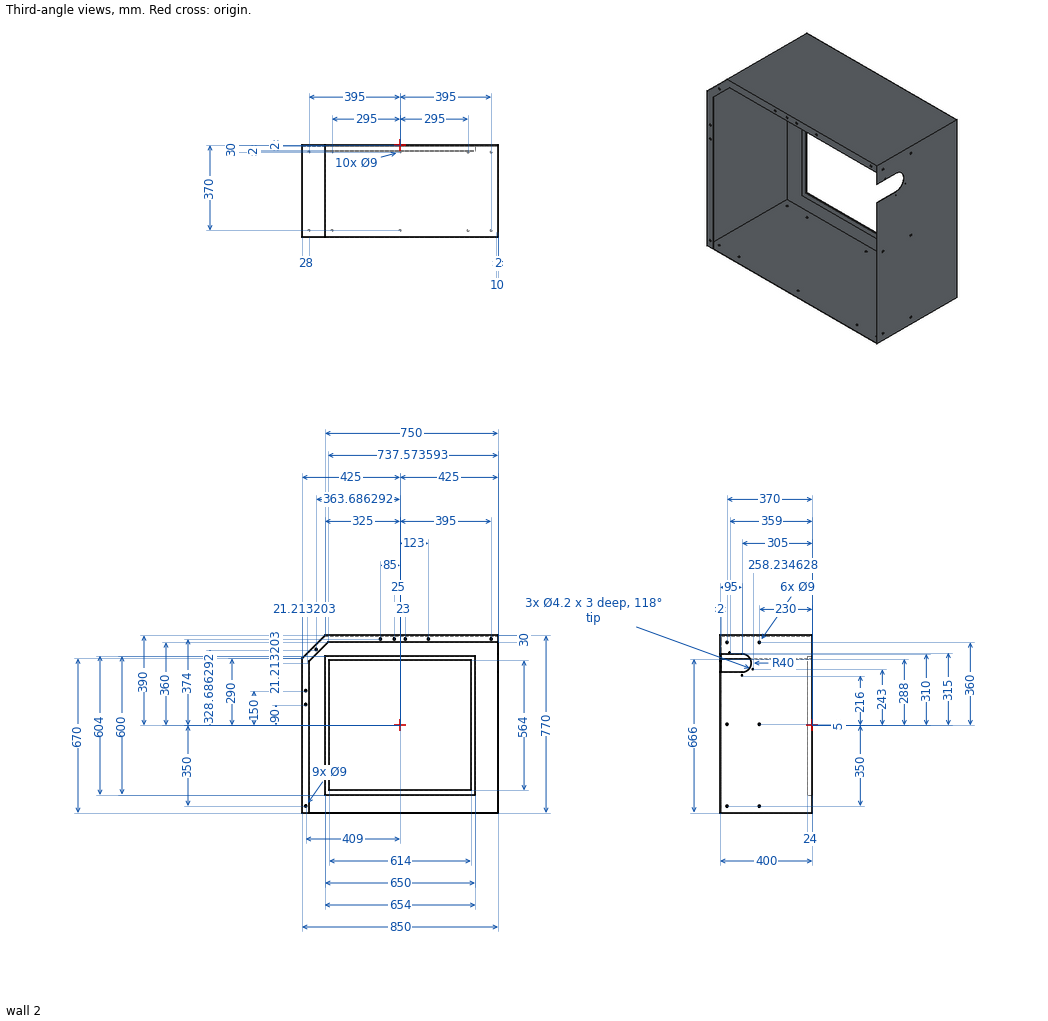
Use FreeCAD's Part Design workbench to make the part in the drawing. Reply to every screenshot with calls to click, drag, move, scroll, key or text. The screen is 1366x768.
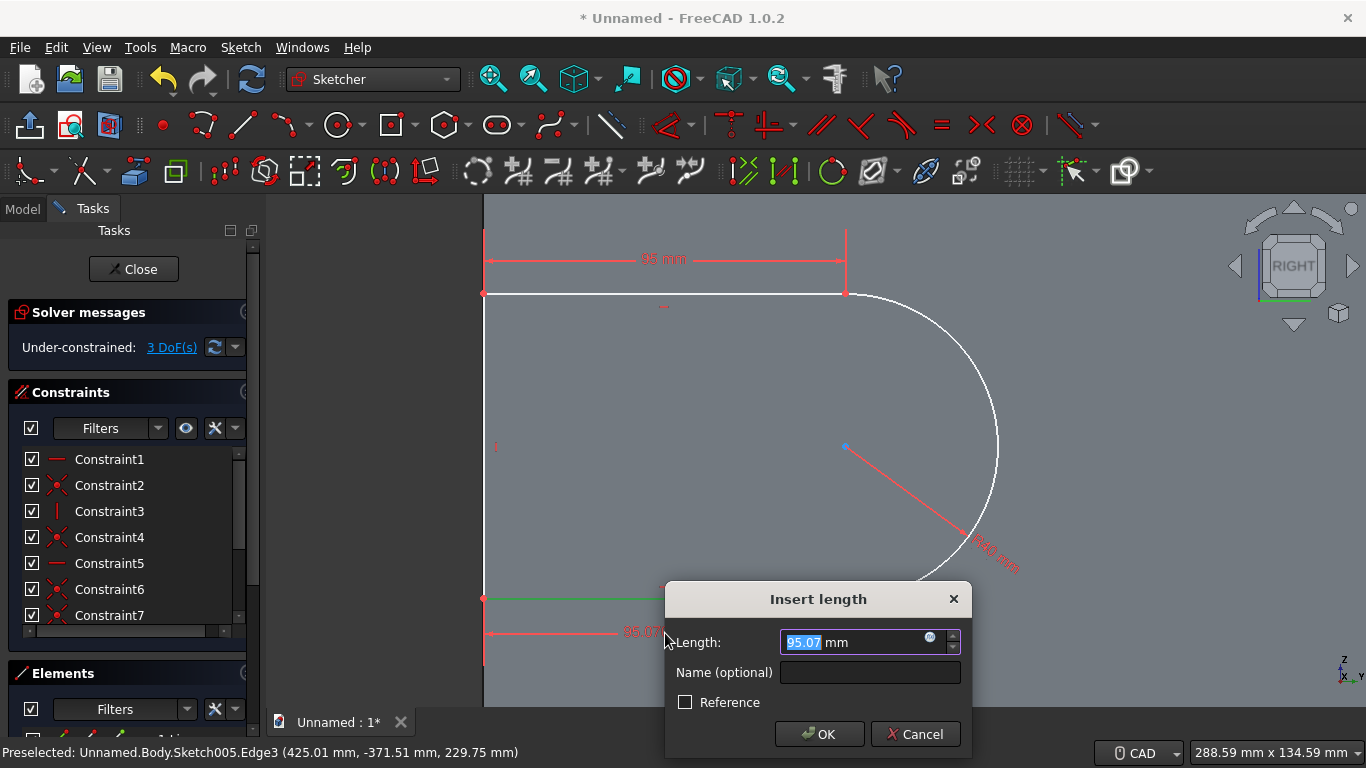
text(95)
key(Return)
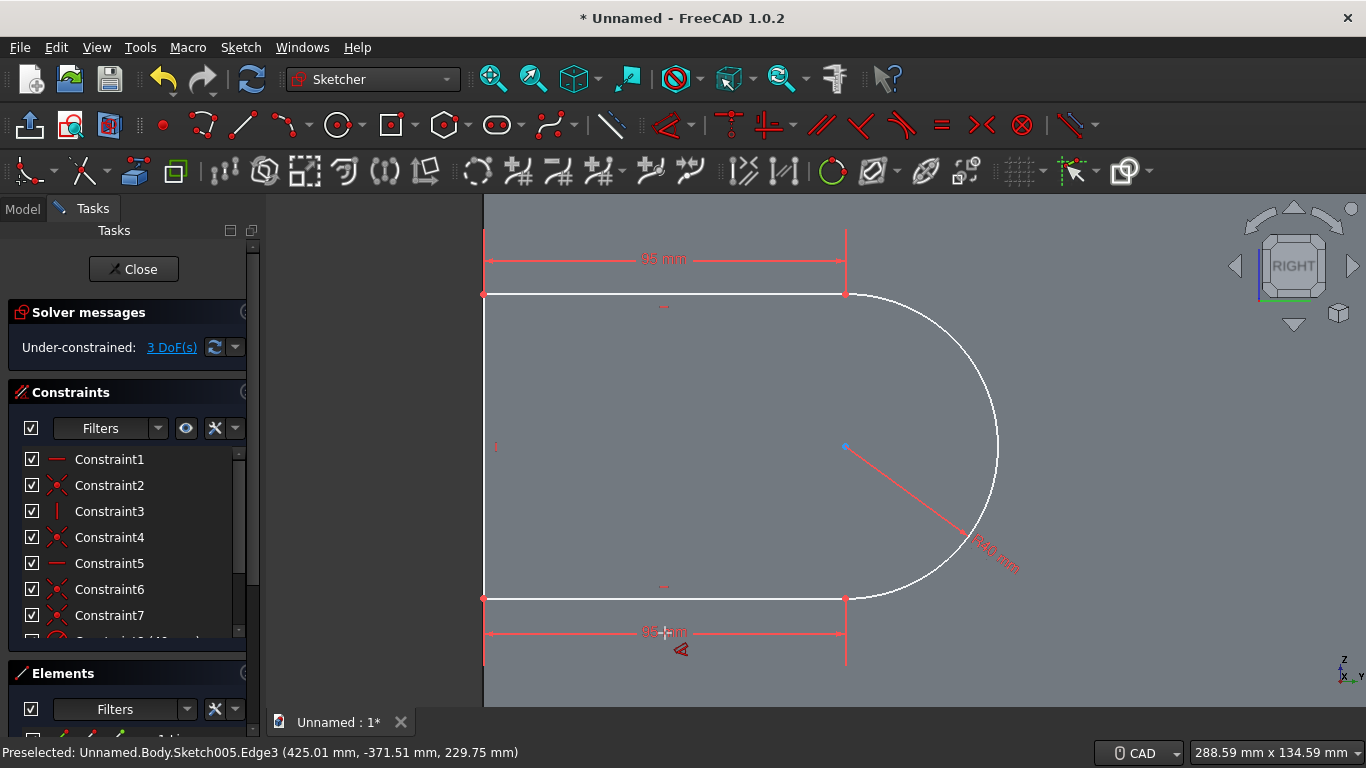
click(846, 294)
click(1023, 260)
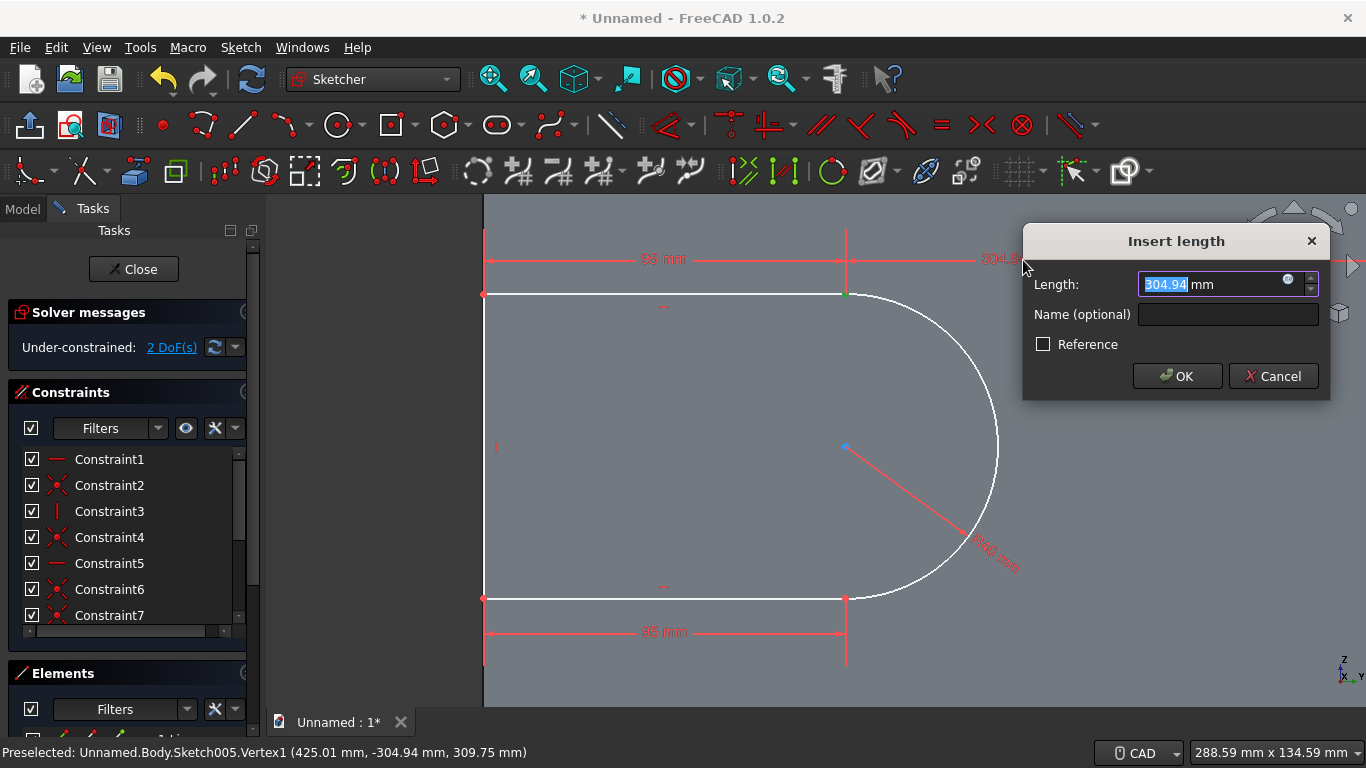
text(305)
key(Return)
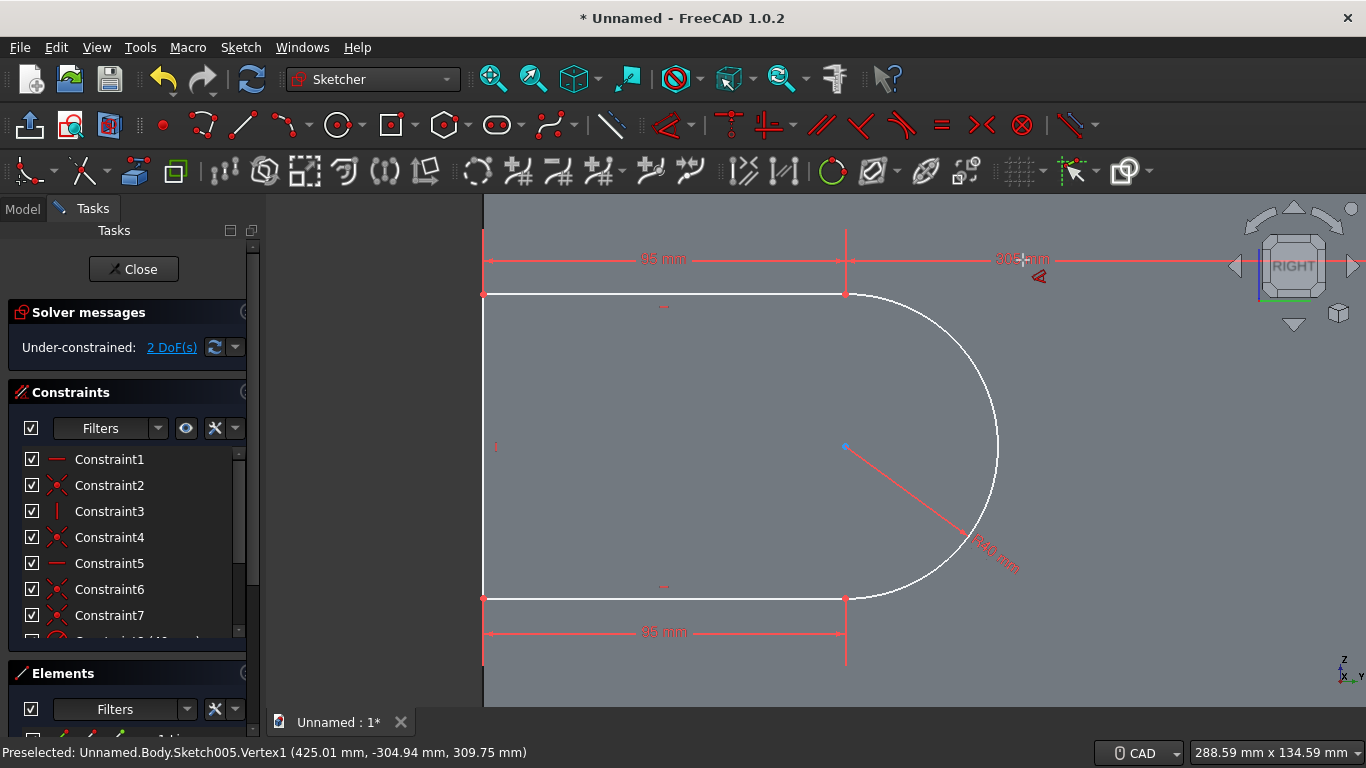
click(846, 294)
click(812, 487)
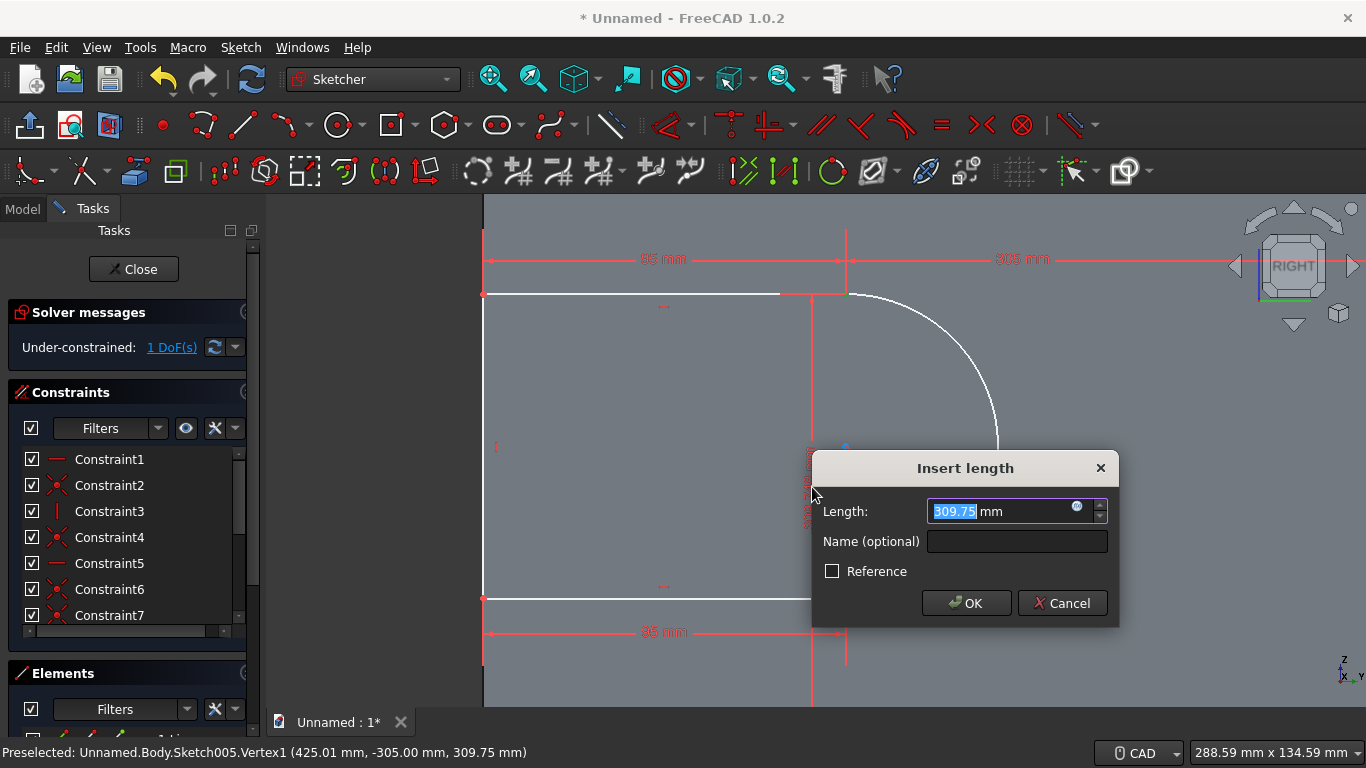
text(310)
key(Return)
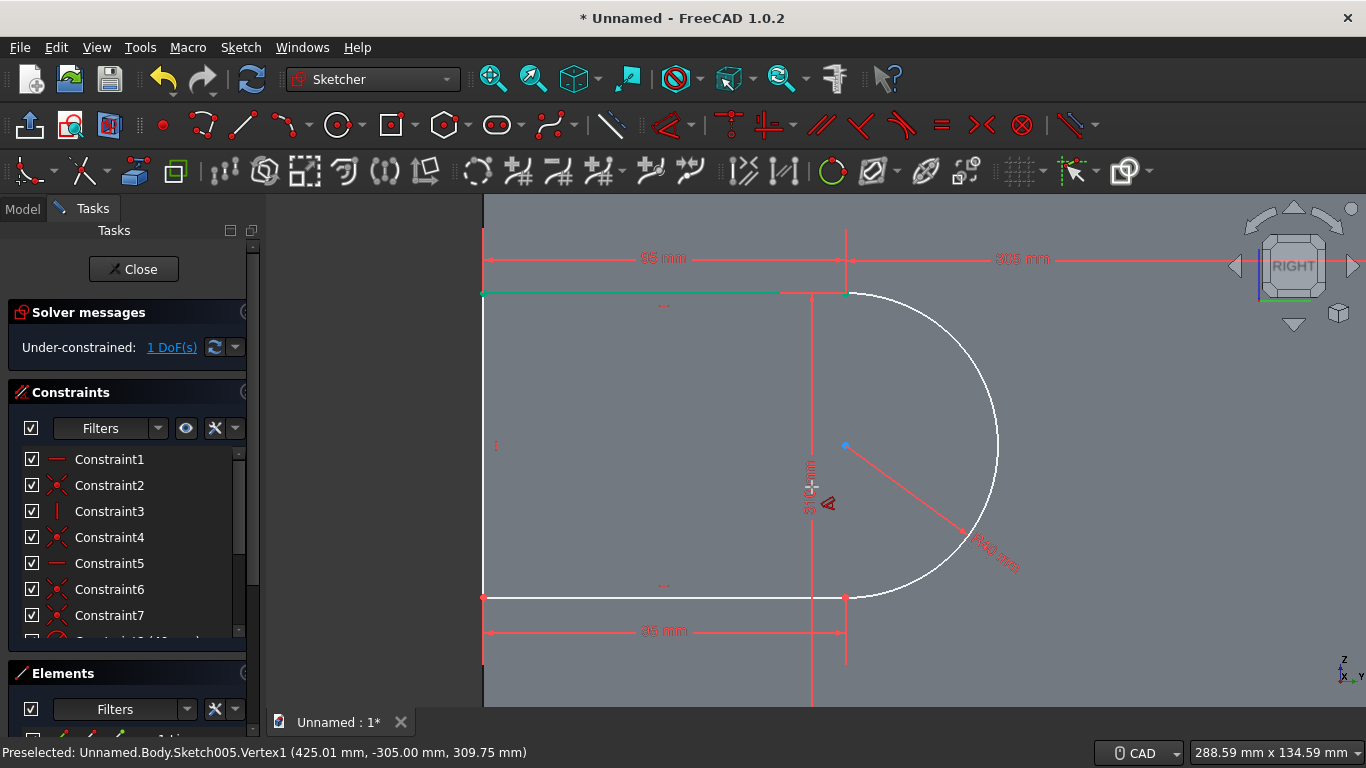
click(845, 446)
click(1023, 412)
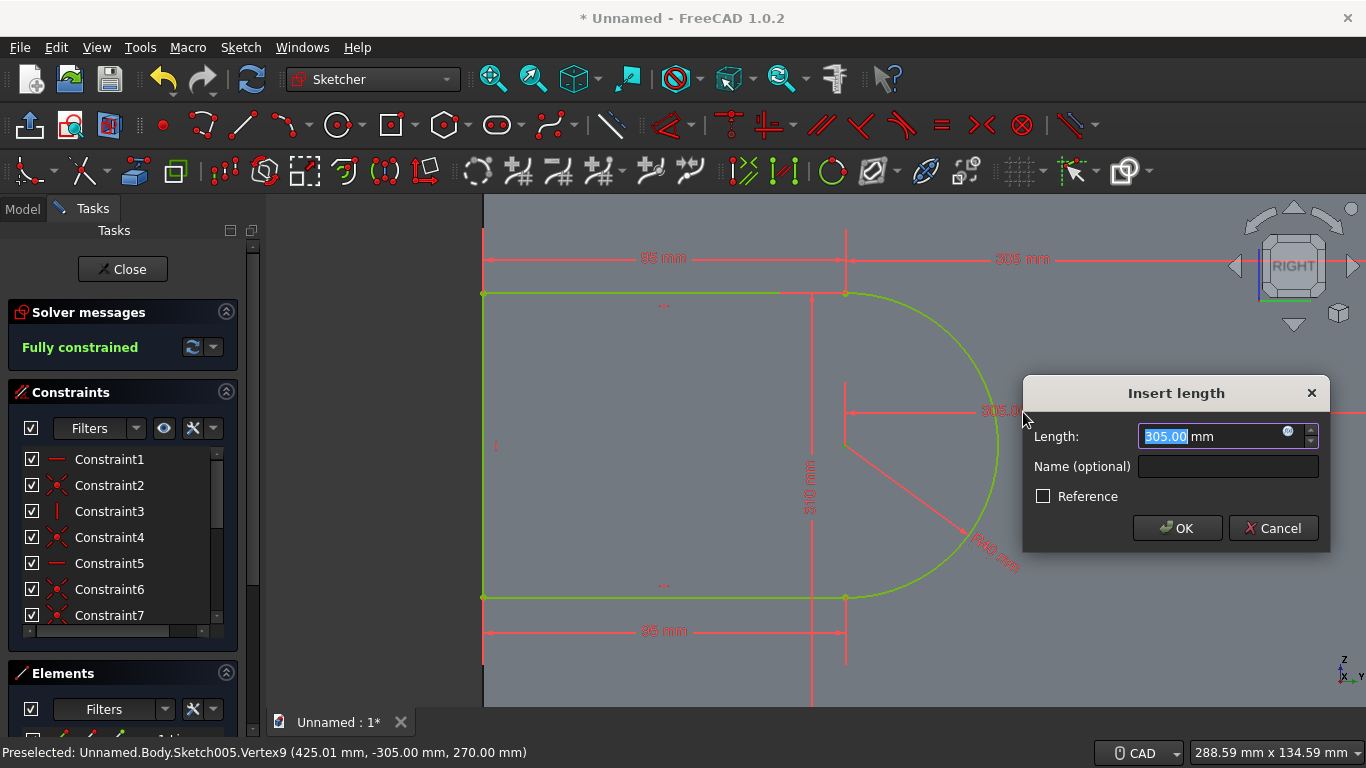
text(305)
key(Return)
key(Escape)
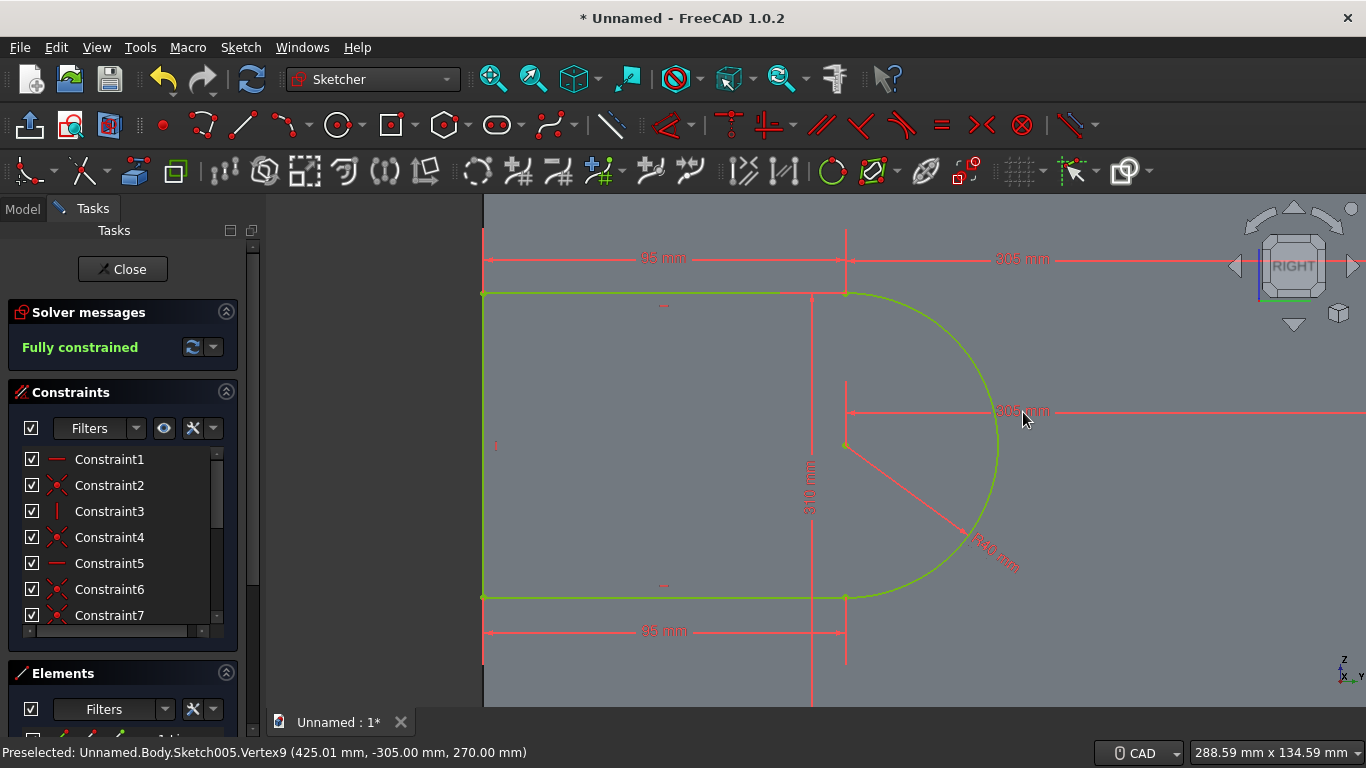
click(123, 269)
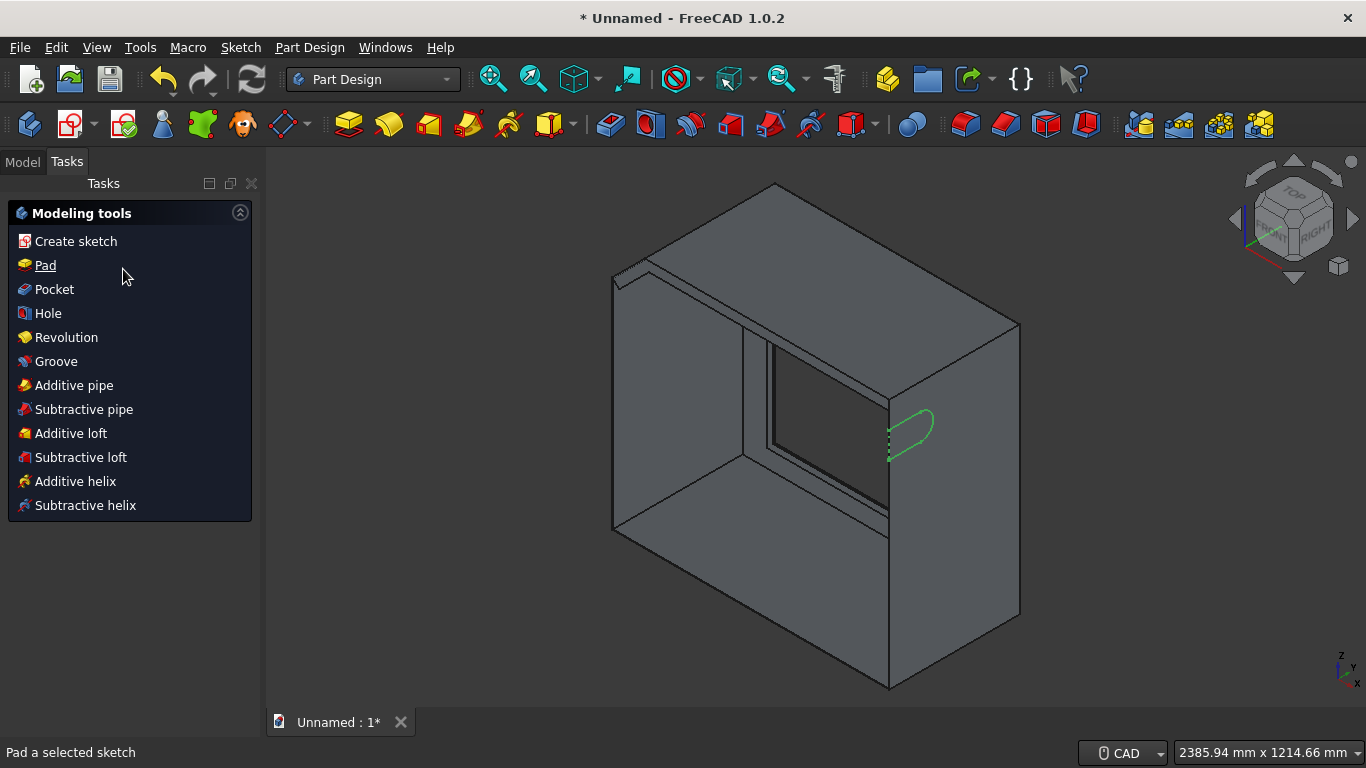
click(612, 124)